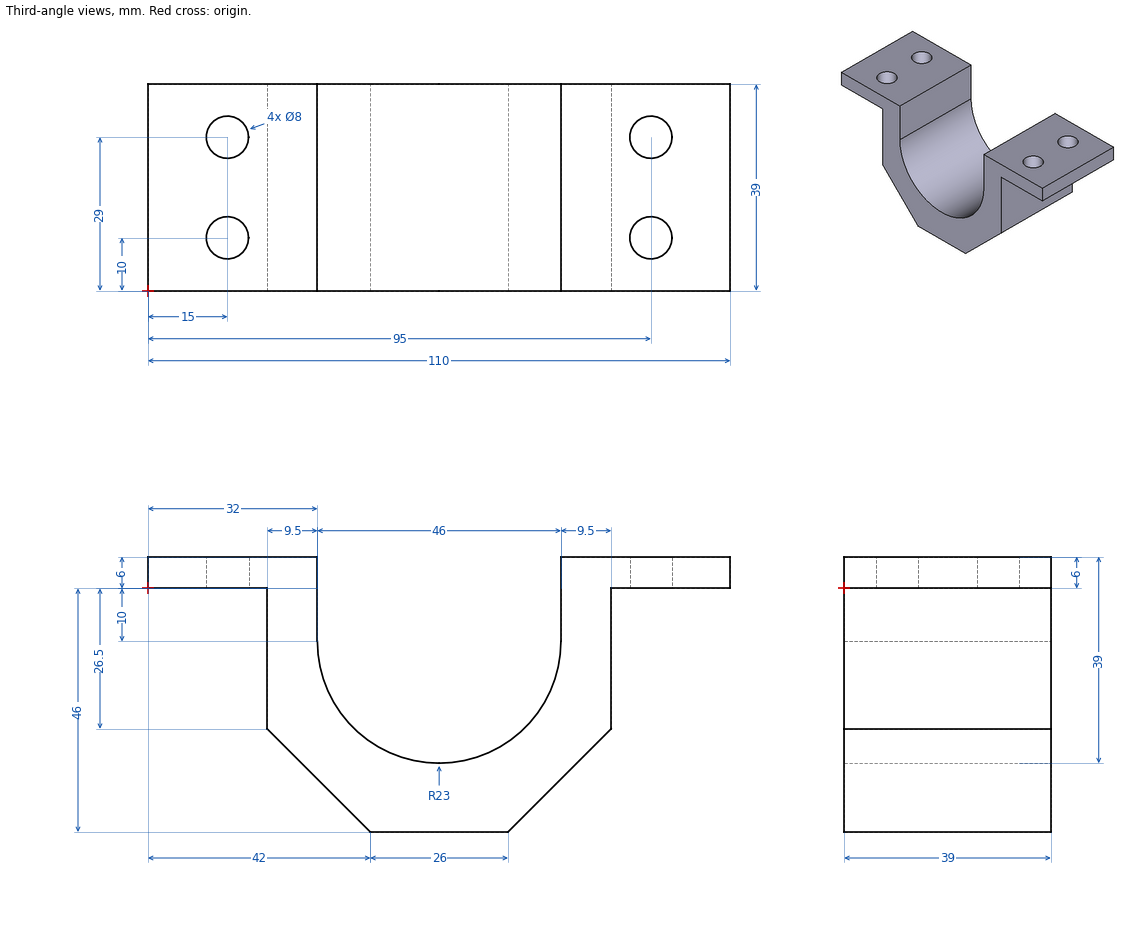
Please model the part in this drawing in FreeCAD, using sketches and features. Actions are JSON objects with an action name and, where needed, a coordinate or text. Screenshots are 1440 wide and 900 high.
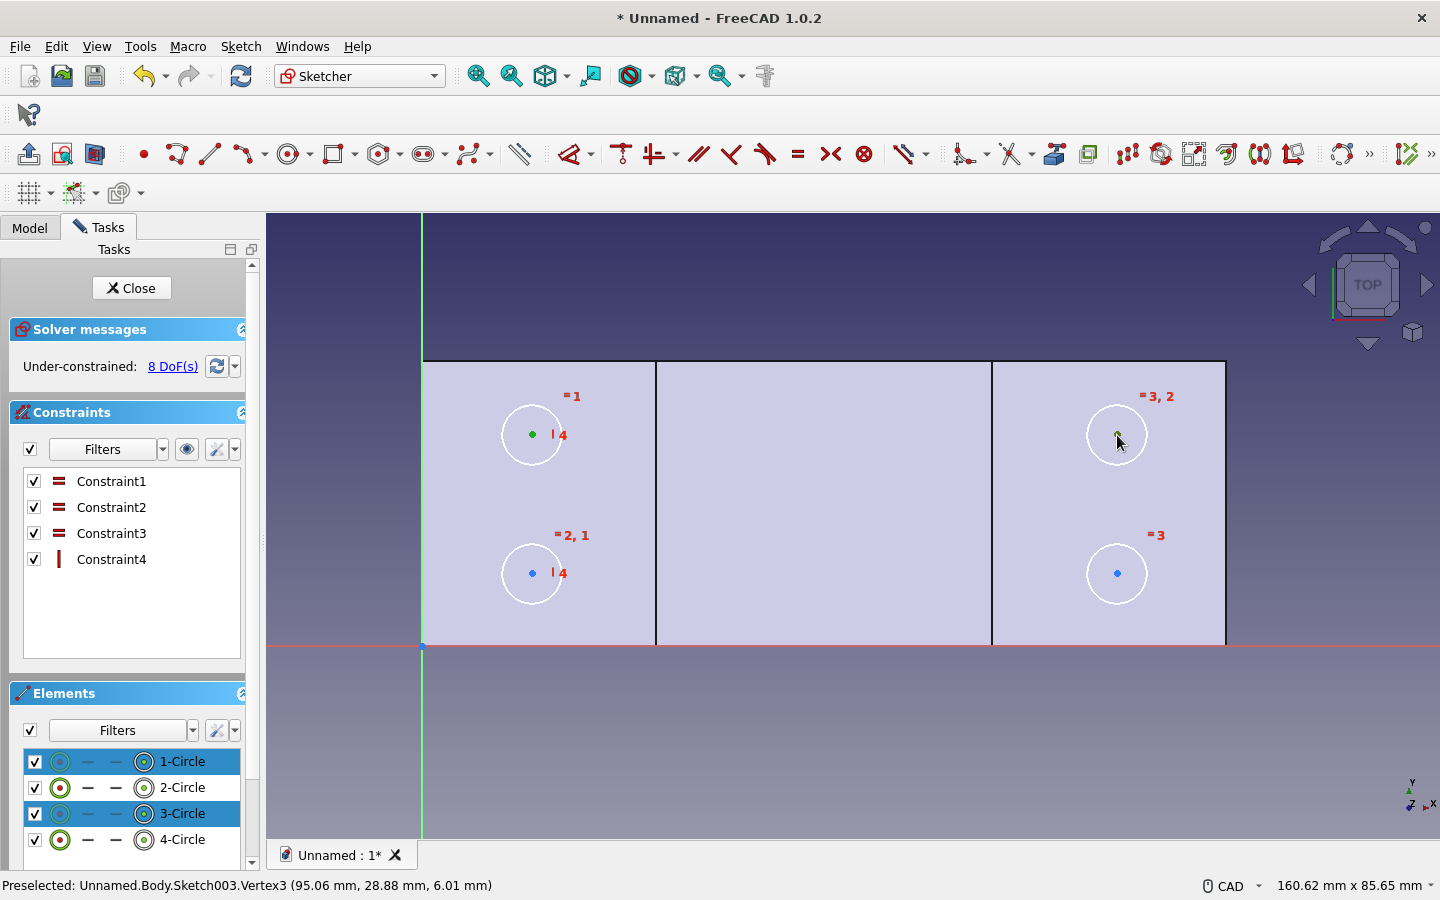
{"action": "key", "text": "h"}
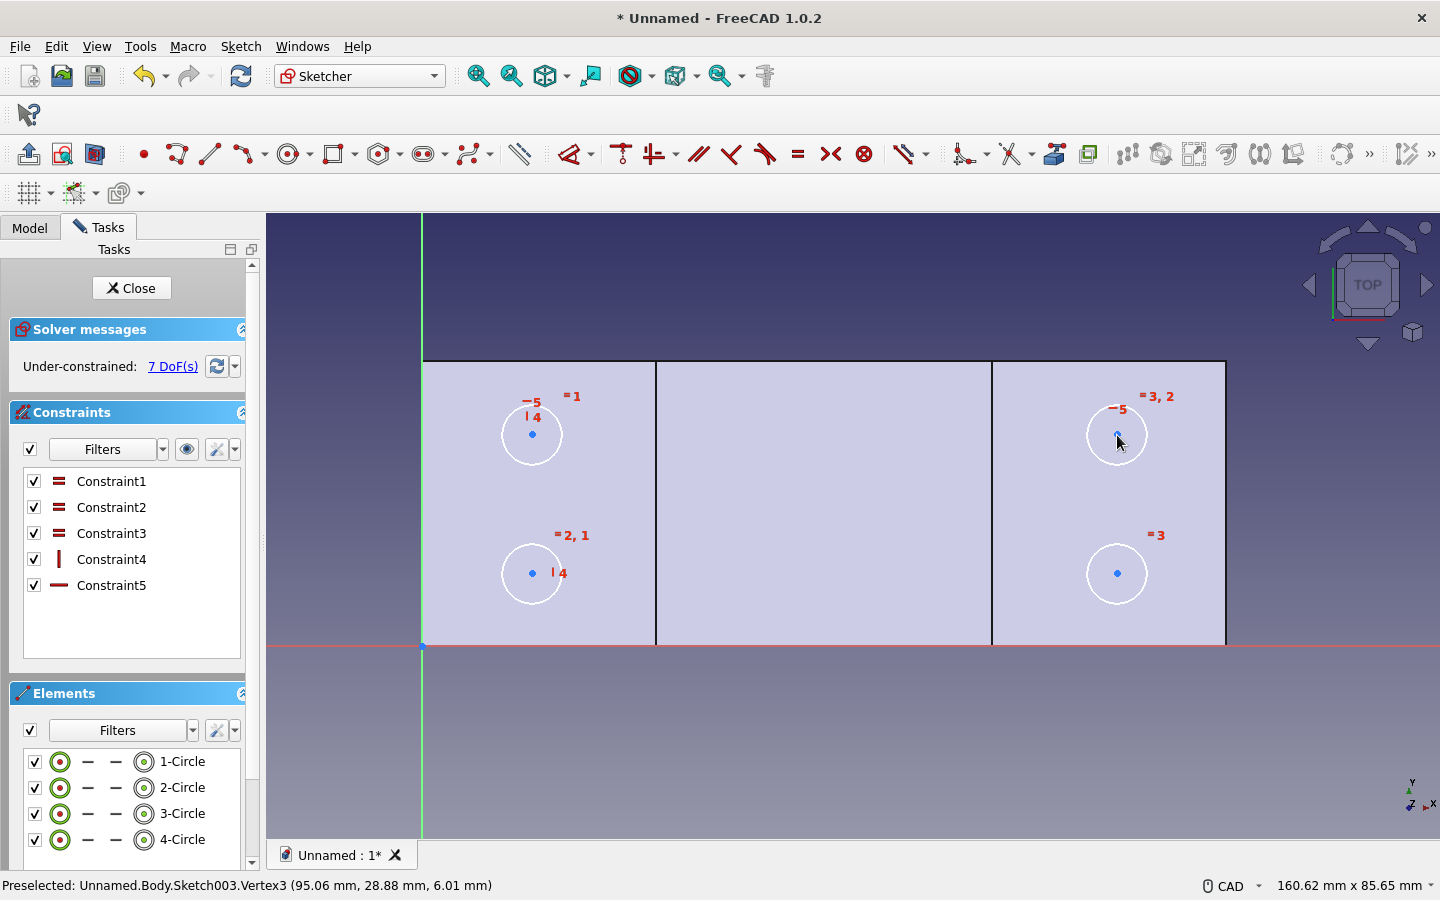
{"action": "left_click", "coordinate": [1117, 435]}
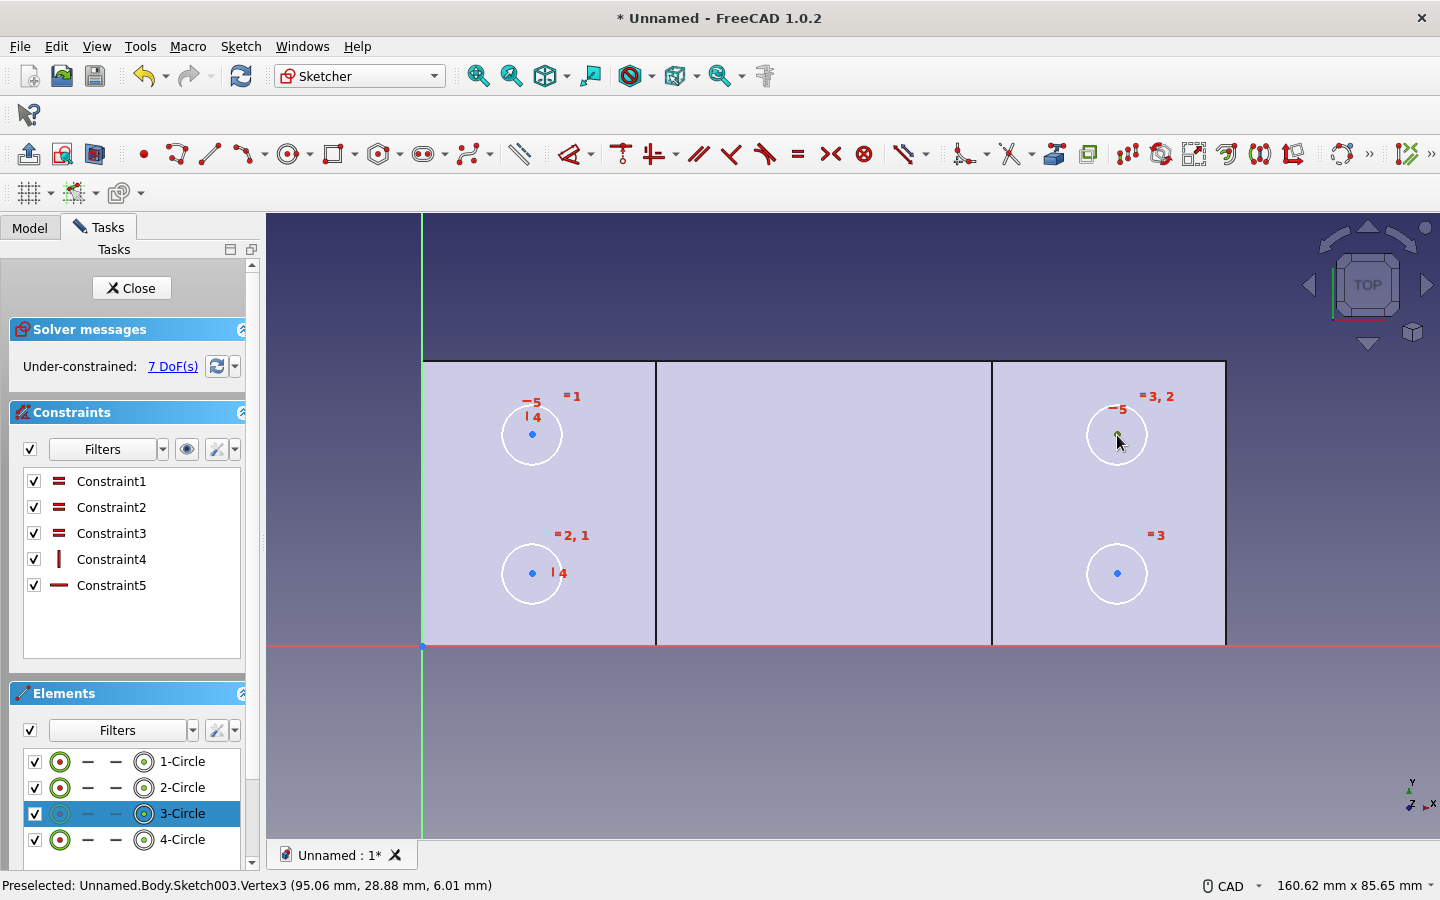
{"action": "left_click", "coordinate": [1117, 574]}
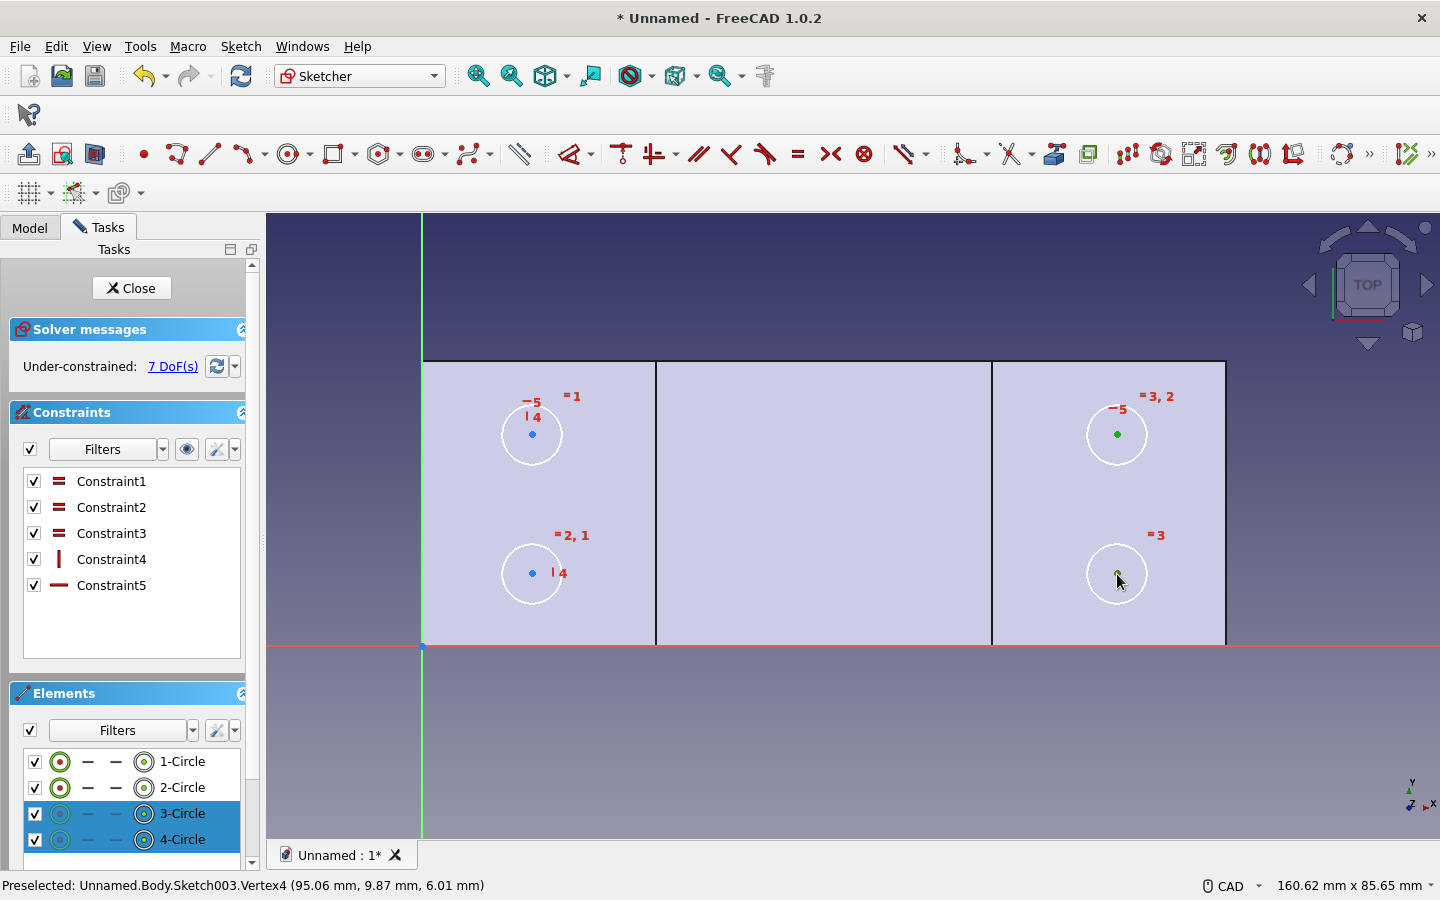
{"action": "key", "text": "v"}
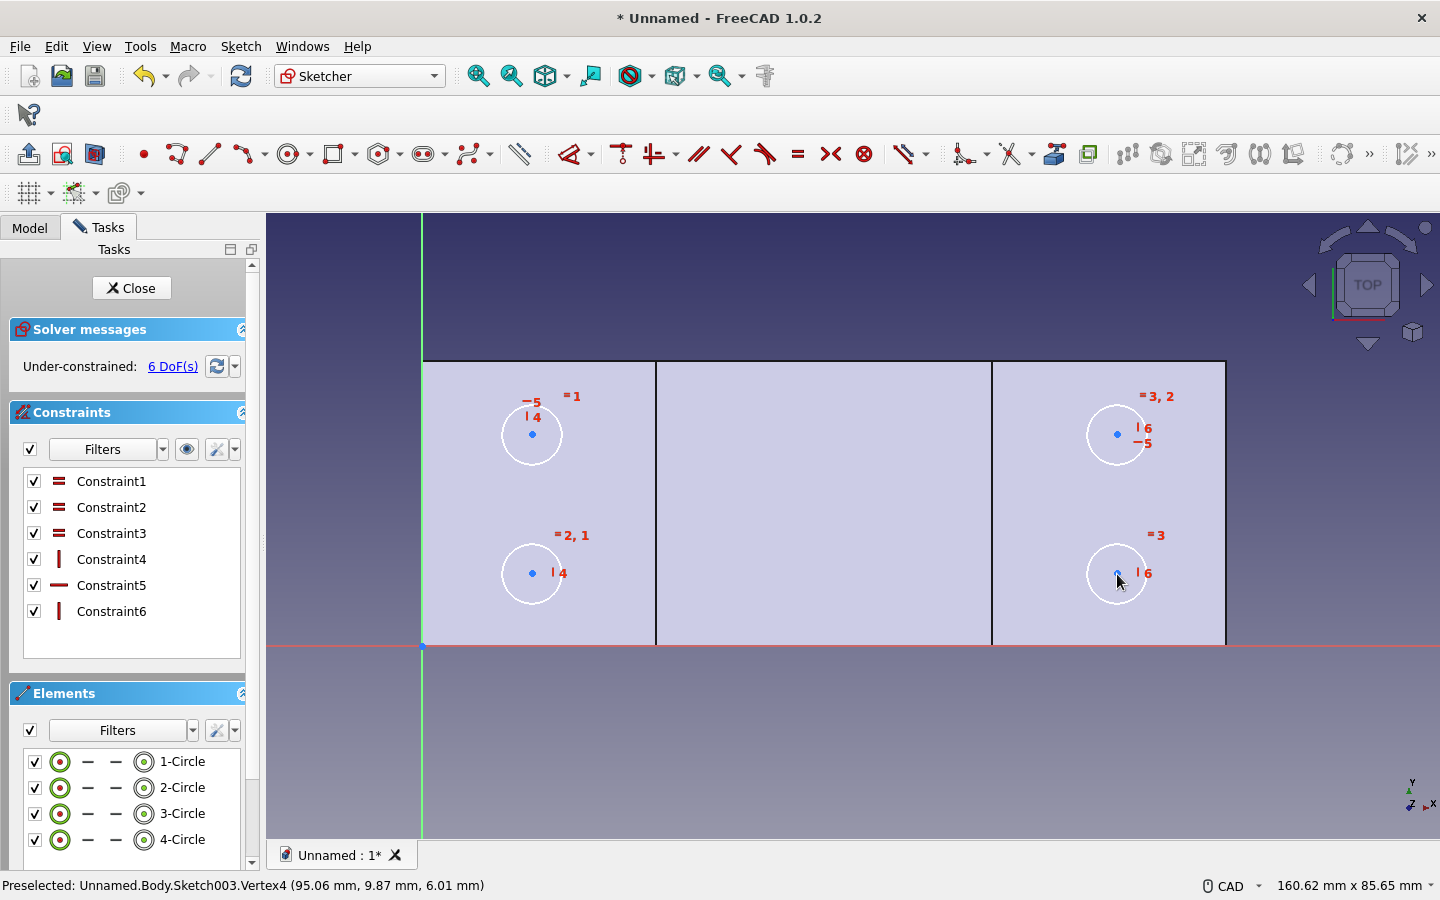
{"action": "left_click", "coordinate": [532, 574]}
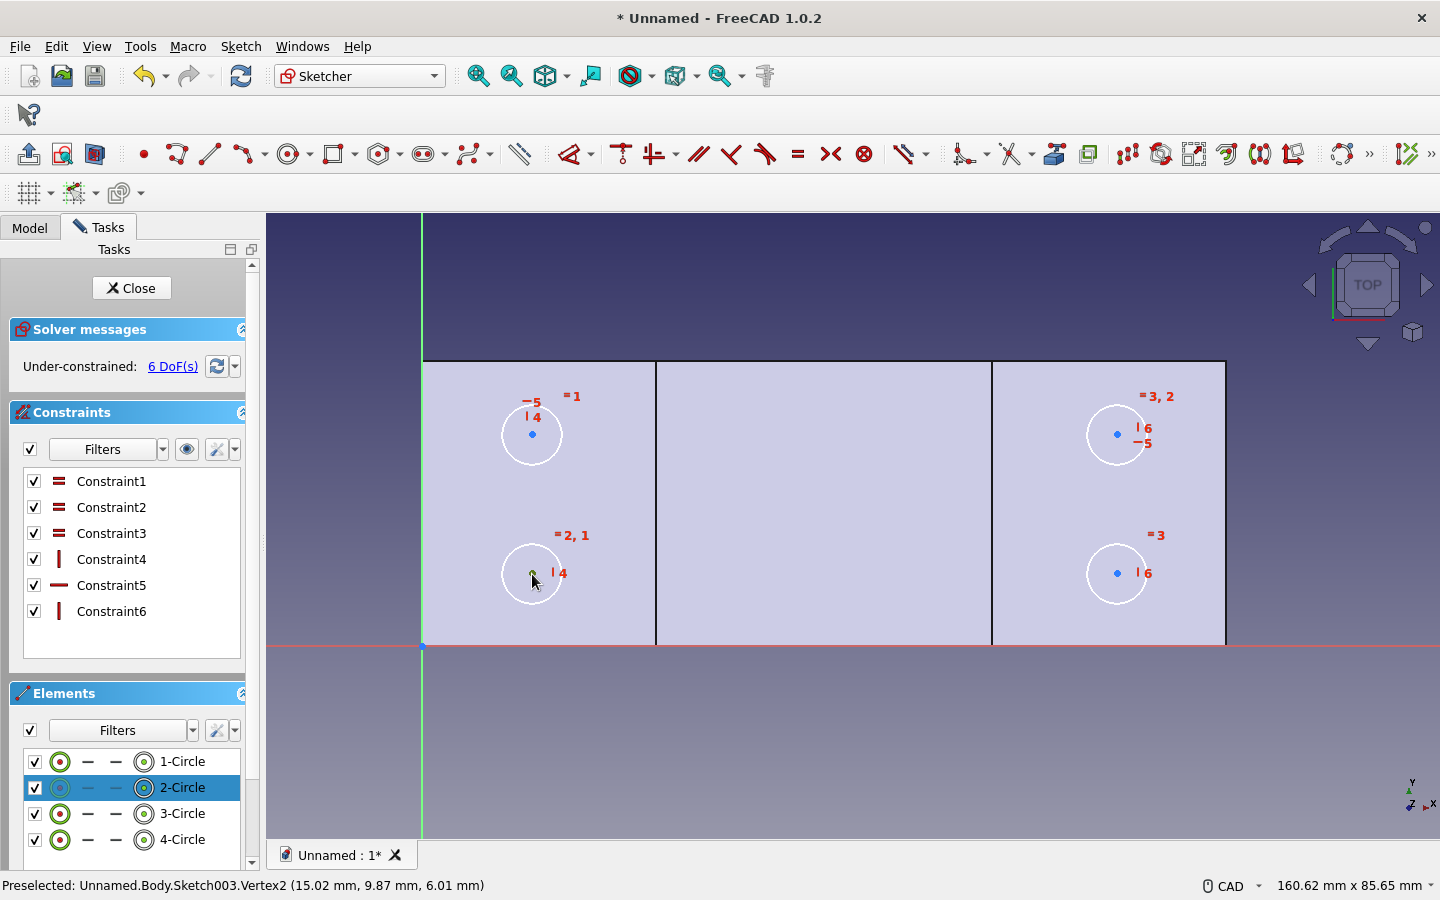
{"action": "left_click", "coordinate": [1117, 574]}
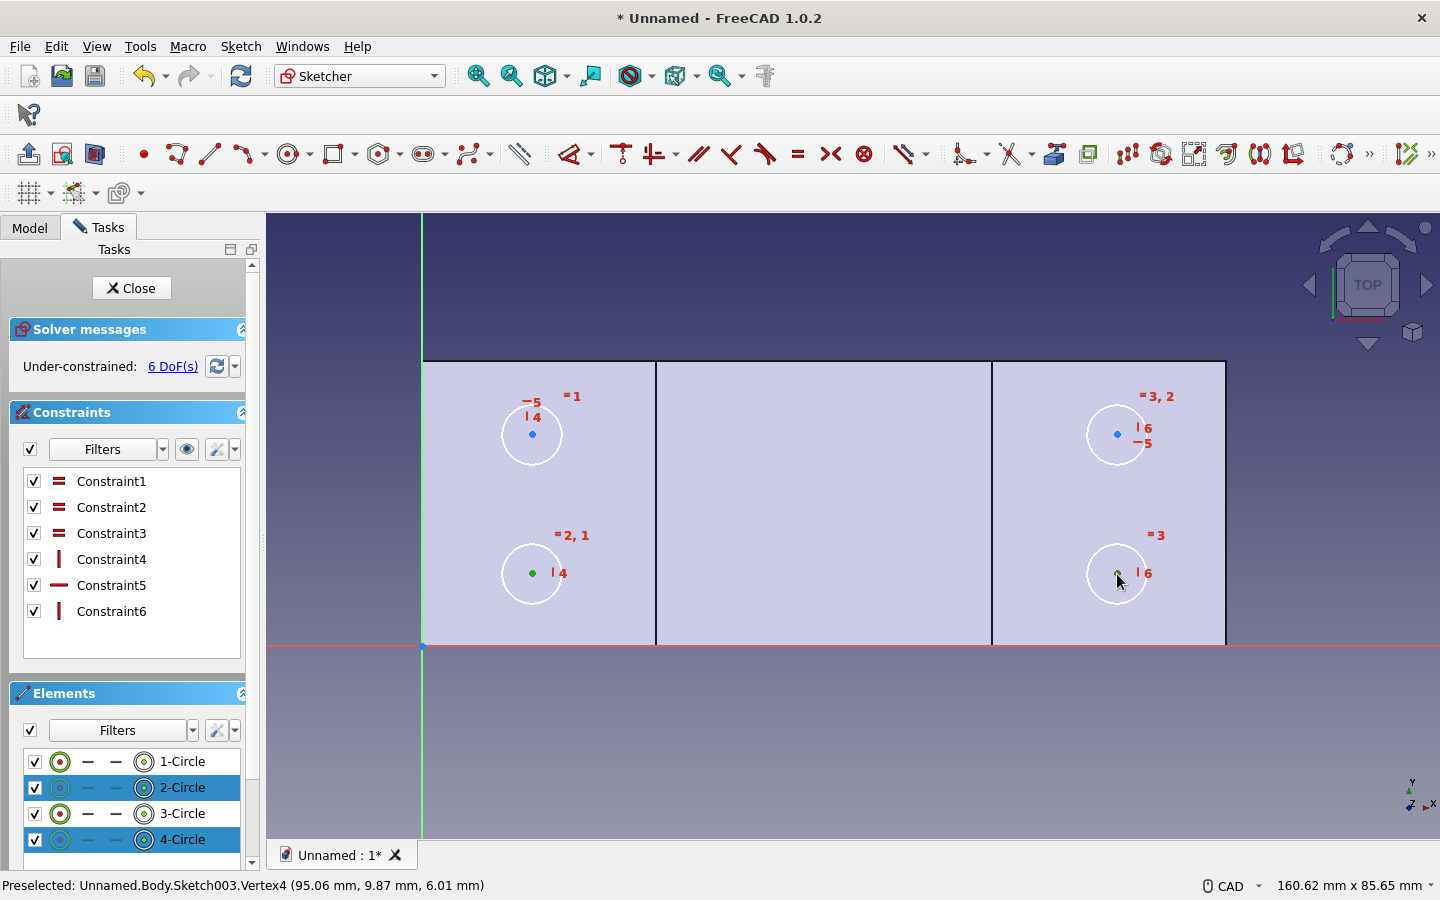
{"action": "key", "text": "h"}